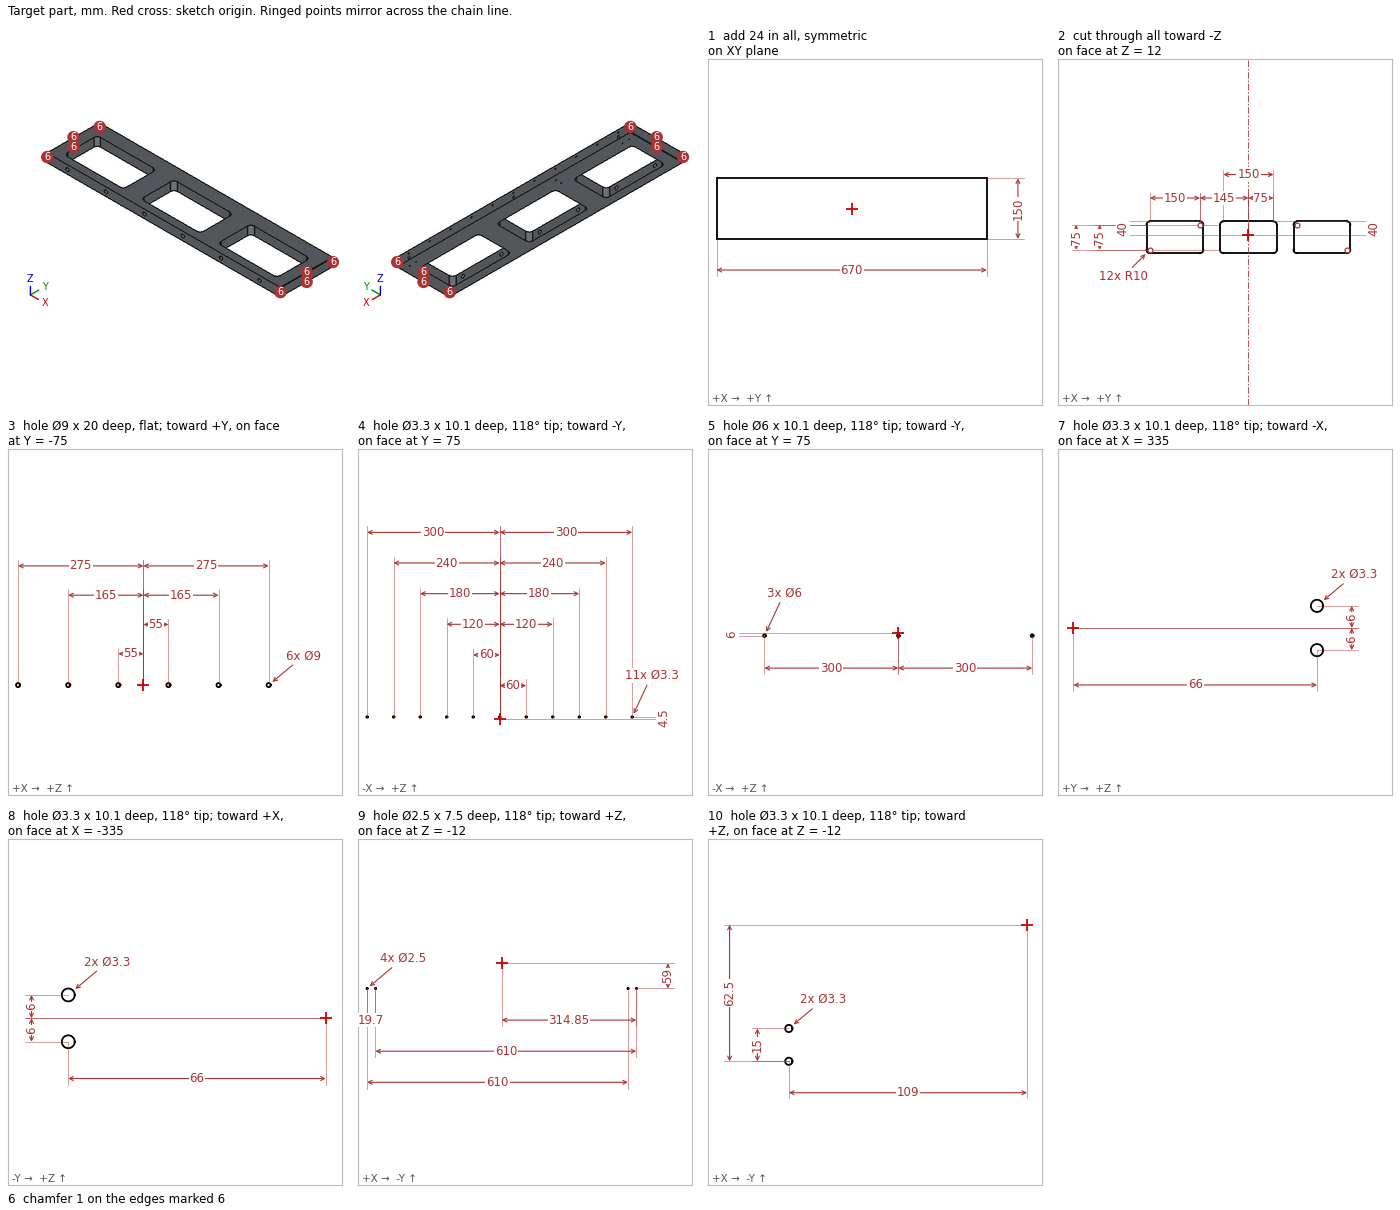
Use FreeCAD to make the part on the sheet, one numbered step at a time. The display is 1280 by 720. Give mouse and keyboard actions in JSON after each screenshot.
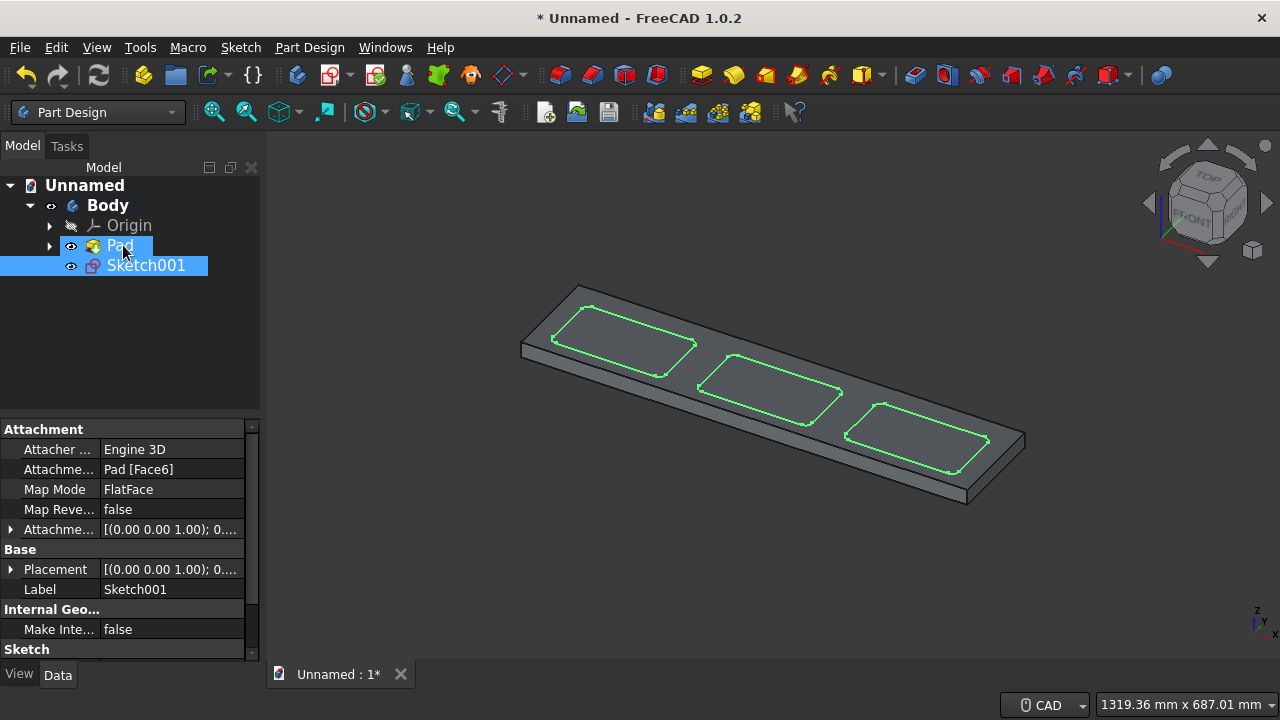
{"action": "left_click", "coordinate": [916, 76]}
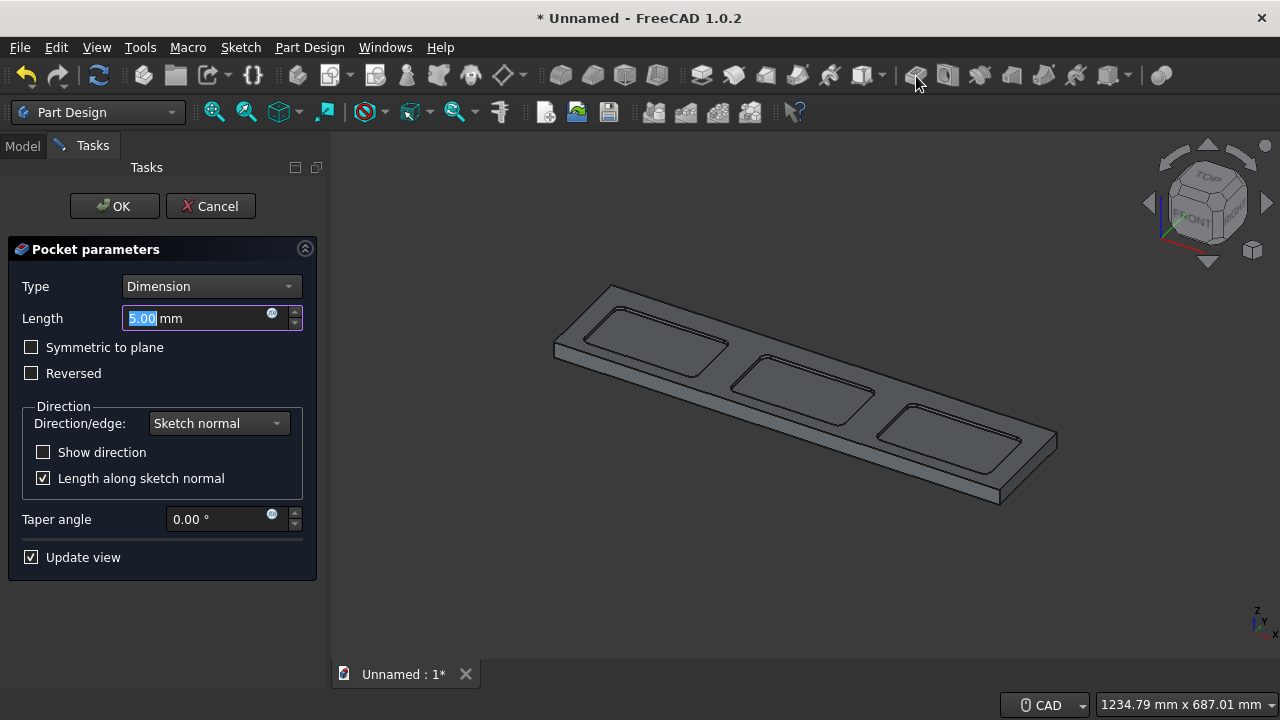
{"action": "left_click", "coordinate": [212, 286]}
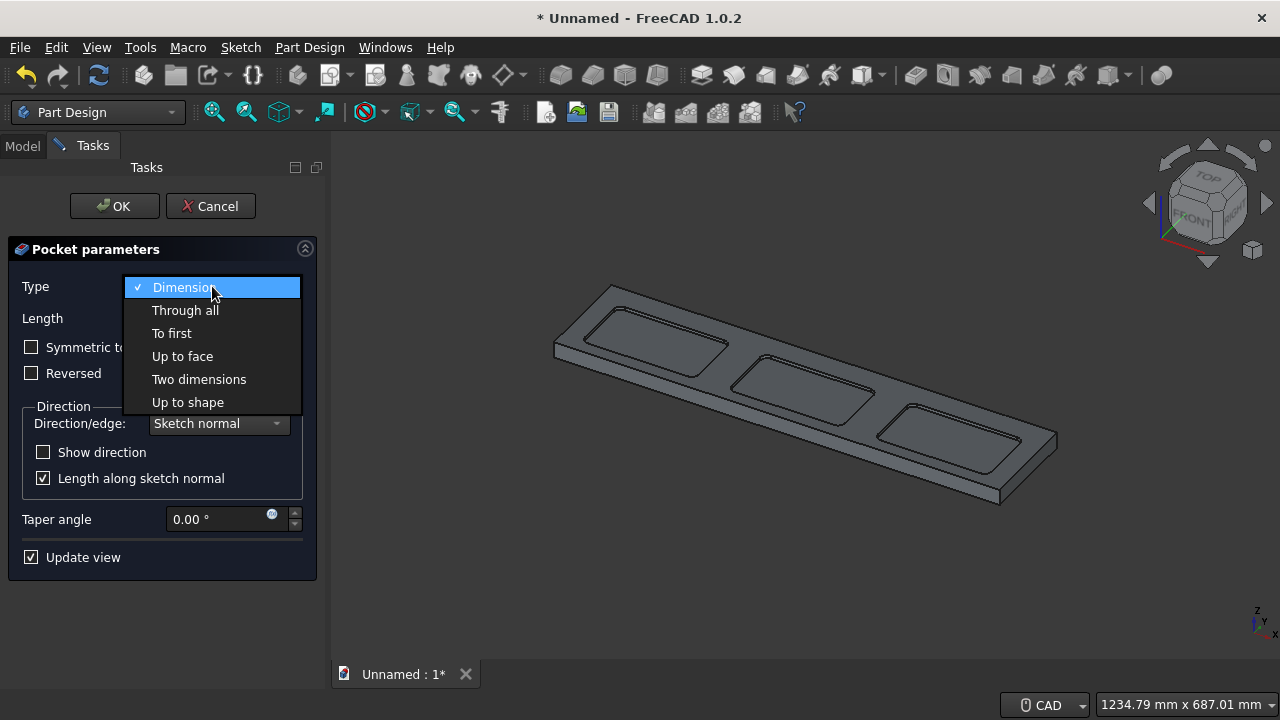
{"action": "left_click", "coordinate": [212, 310]}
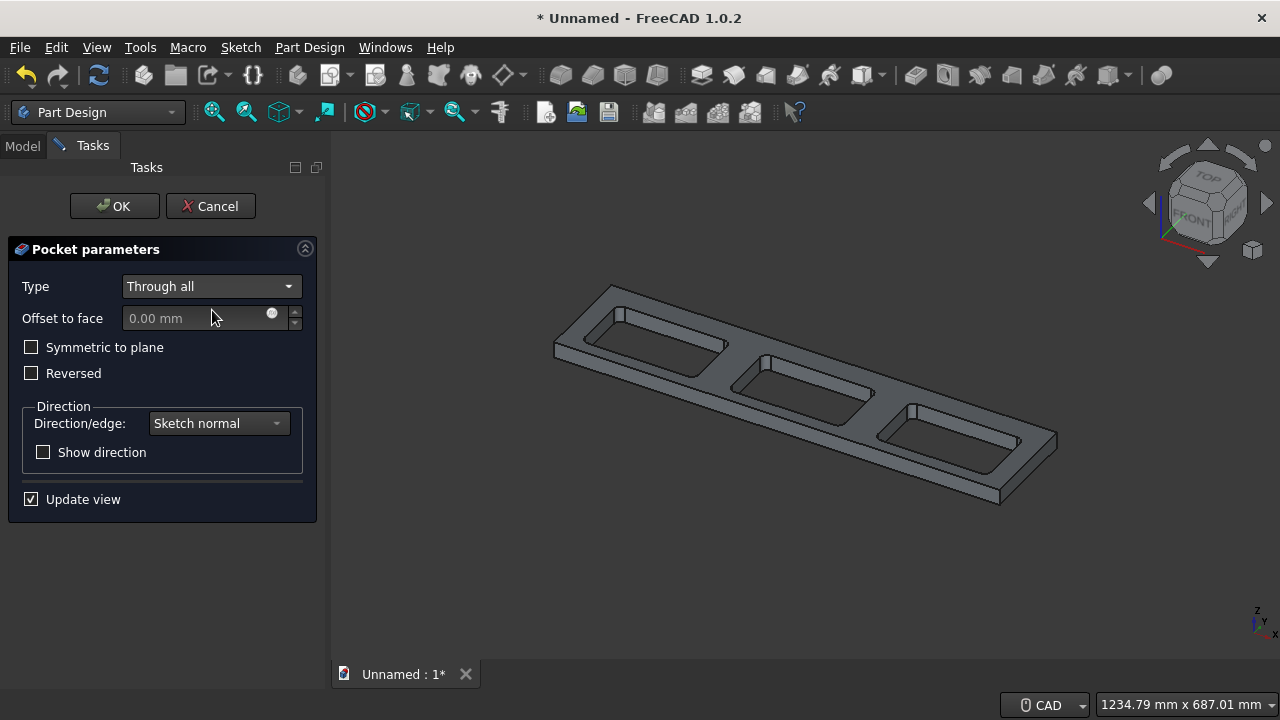
{"action": "left_click", "coordinate": [115, 206]}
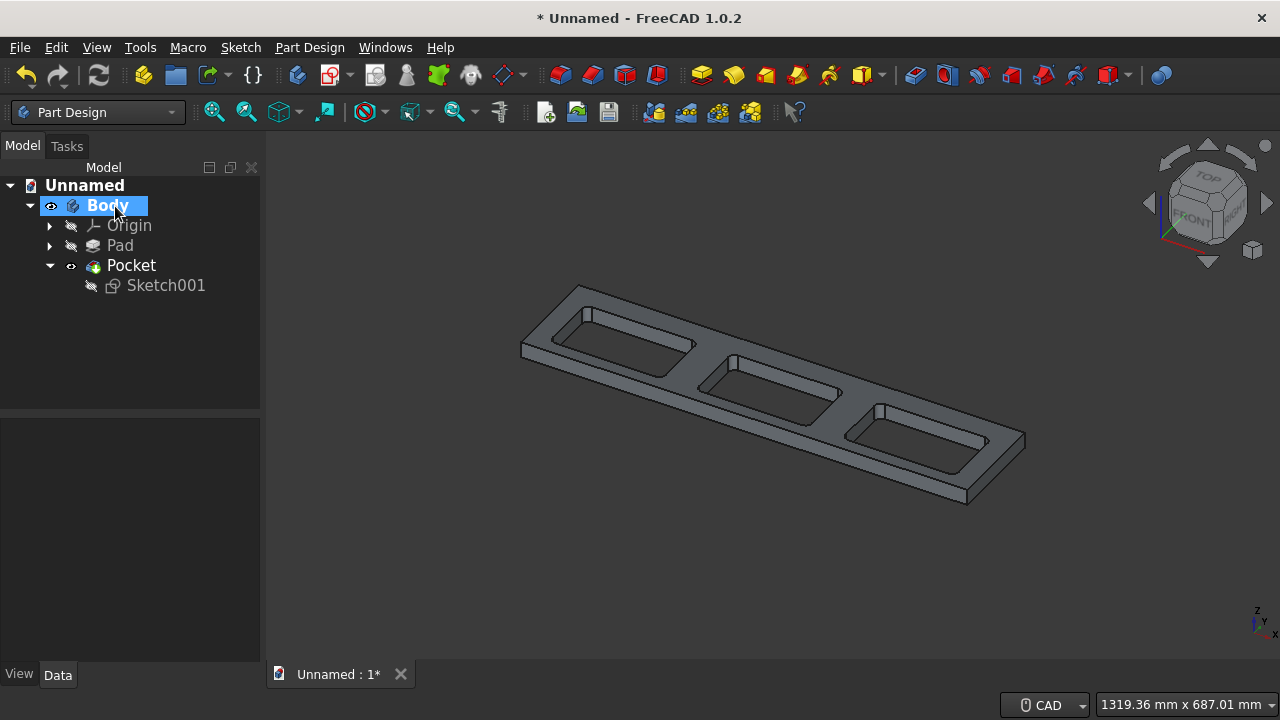
{"action": "key", "text": "0"}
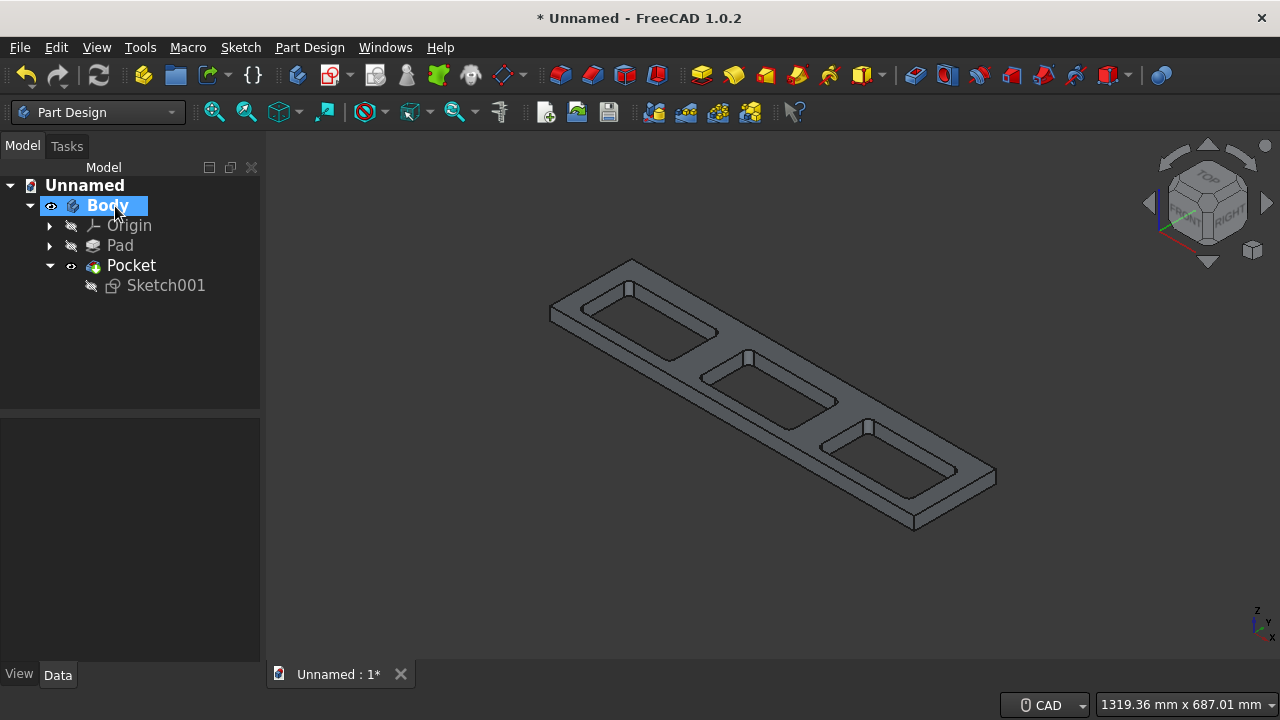
{"action": "key", "text": "1"}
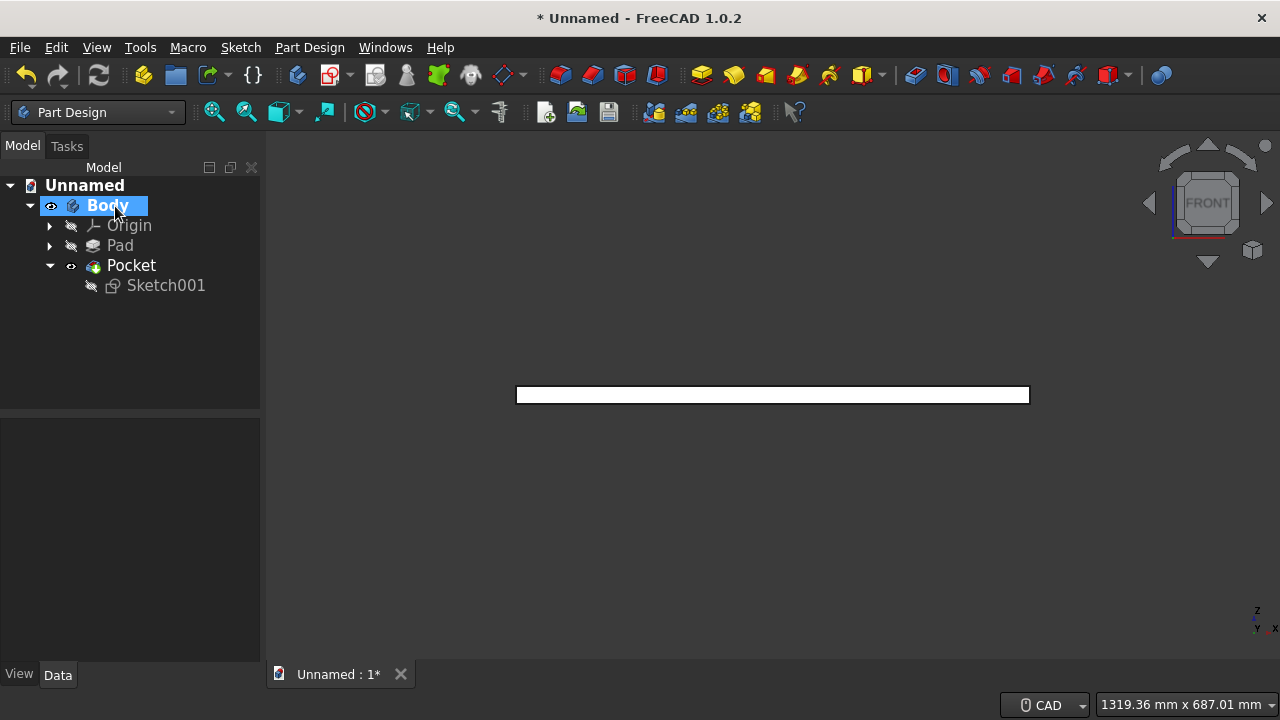
{"action": "left_click", "coordinate": [994, 394]}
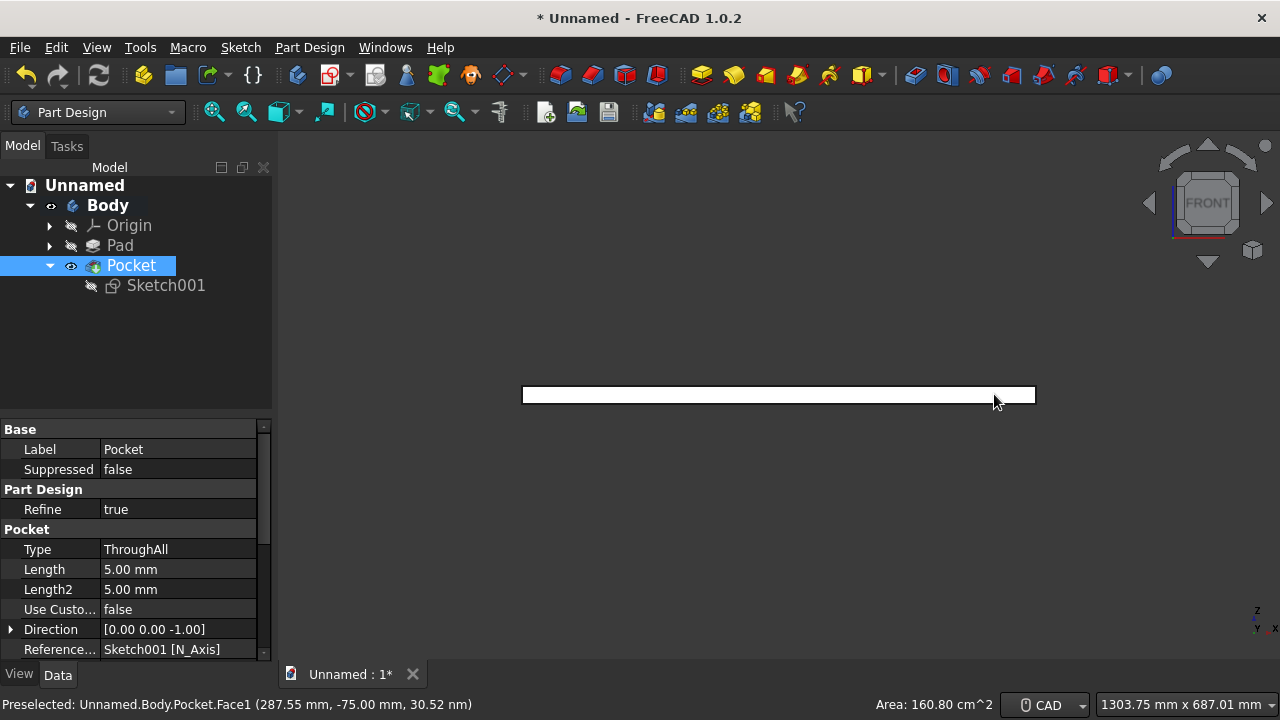
{"action": "left_click", "coordinate": [330, 76]}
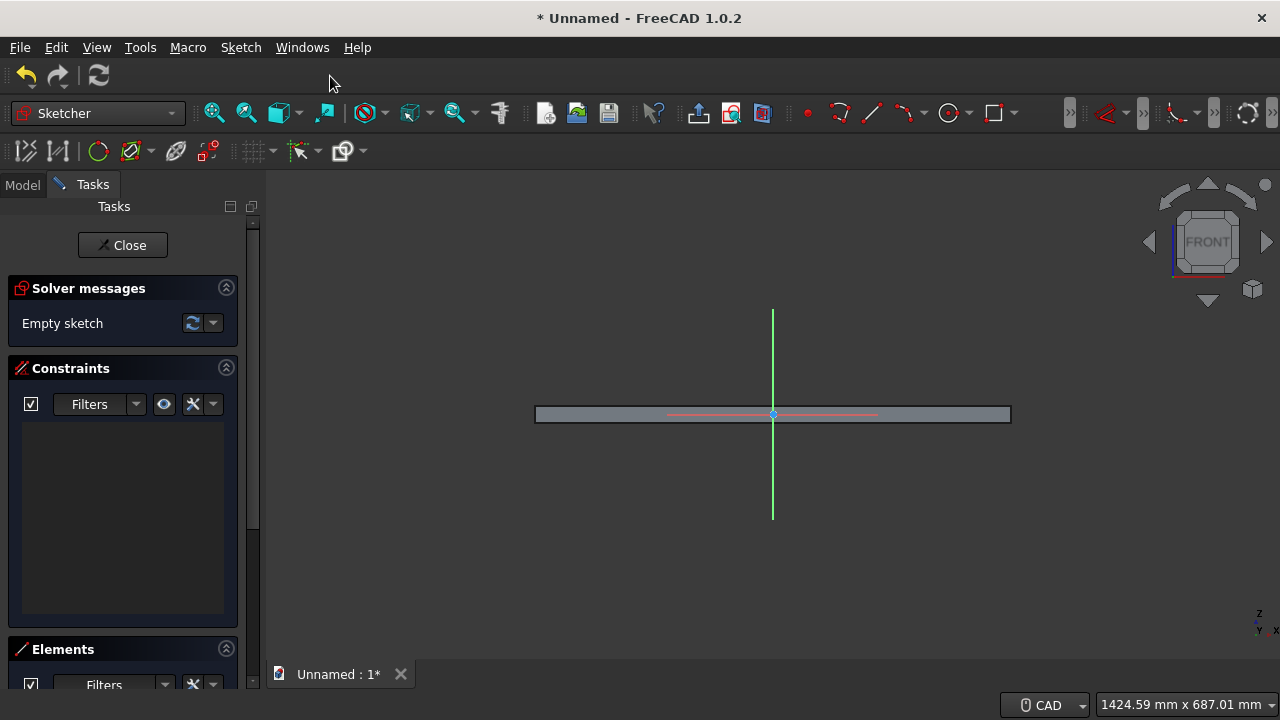
{"action": "scroll", "coordinate": [912, 415], "scroll_direction": "up", "scroll_amount": 2}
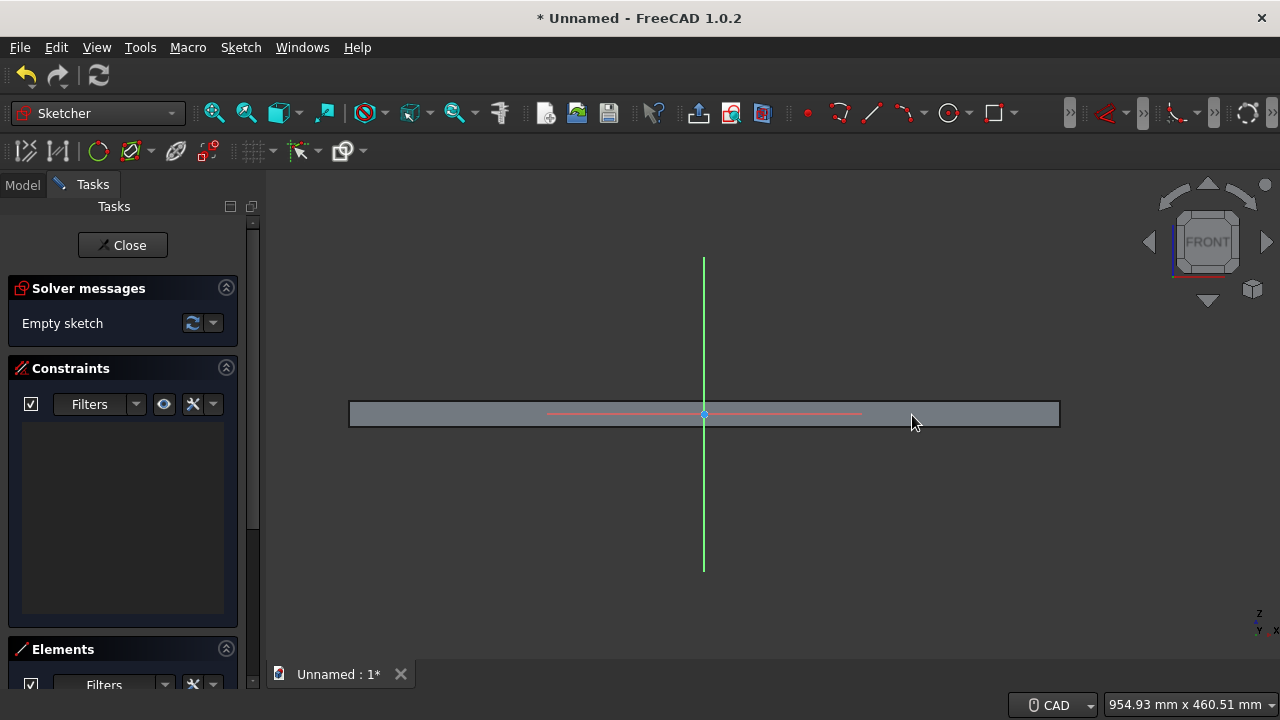
{"action": "left_click", "coordinate": [950, 114]}